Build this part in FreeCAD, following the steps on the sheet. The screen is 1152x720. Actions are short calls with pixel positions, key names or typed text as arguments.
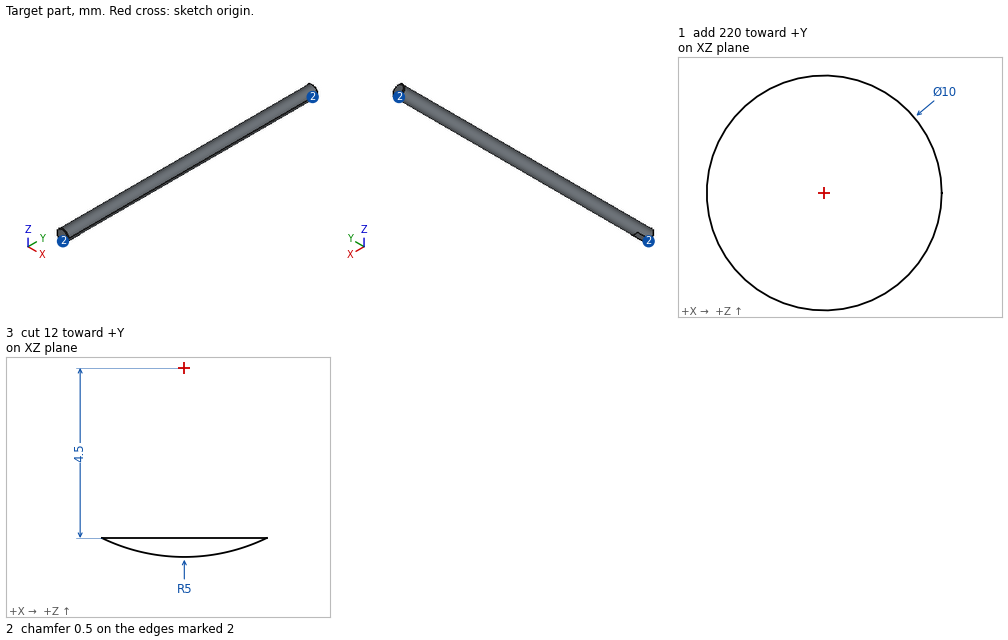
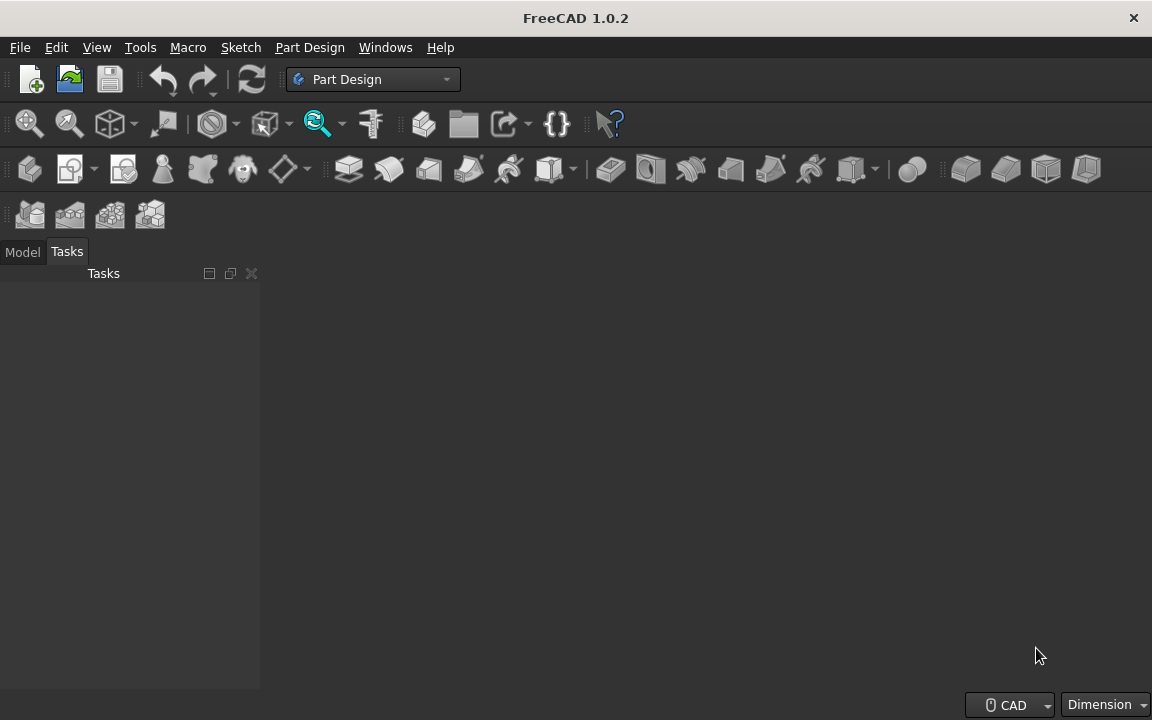
click(30, 80)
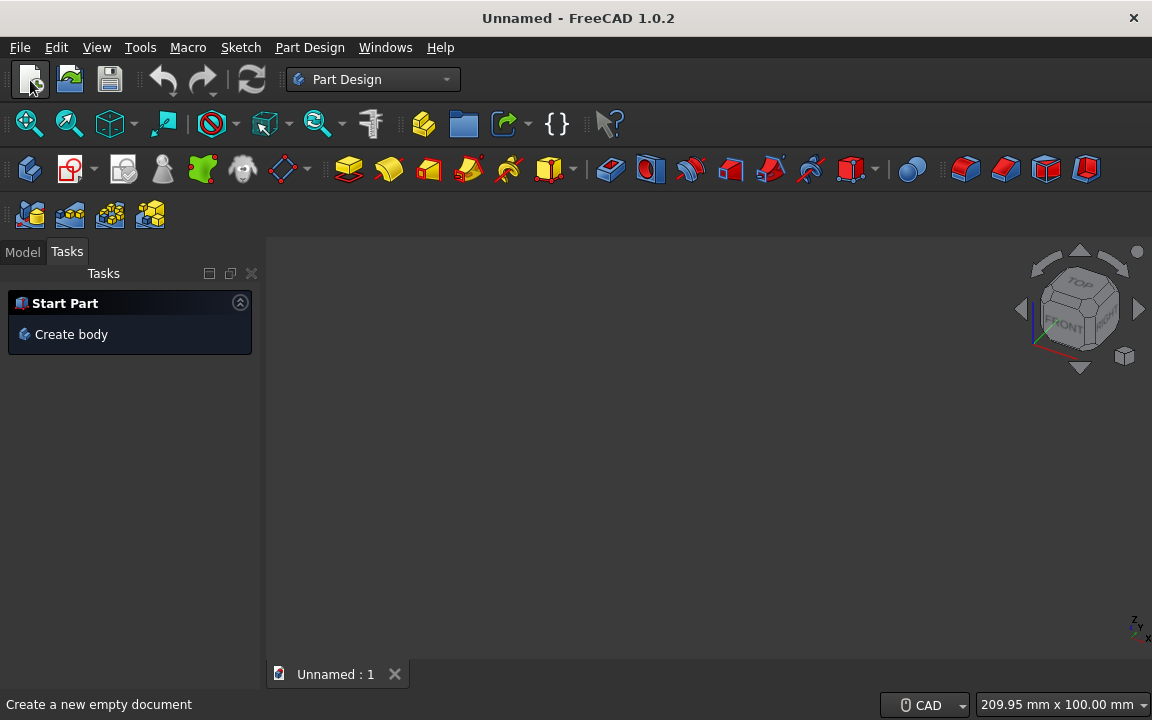
click(70, 170)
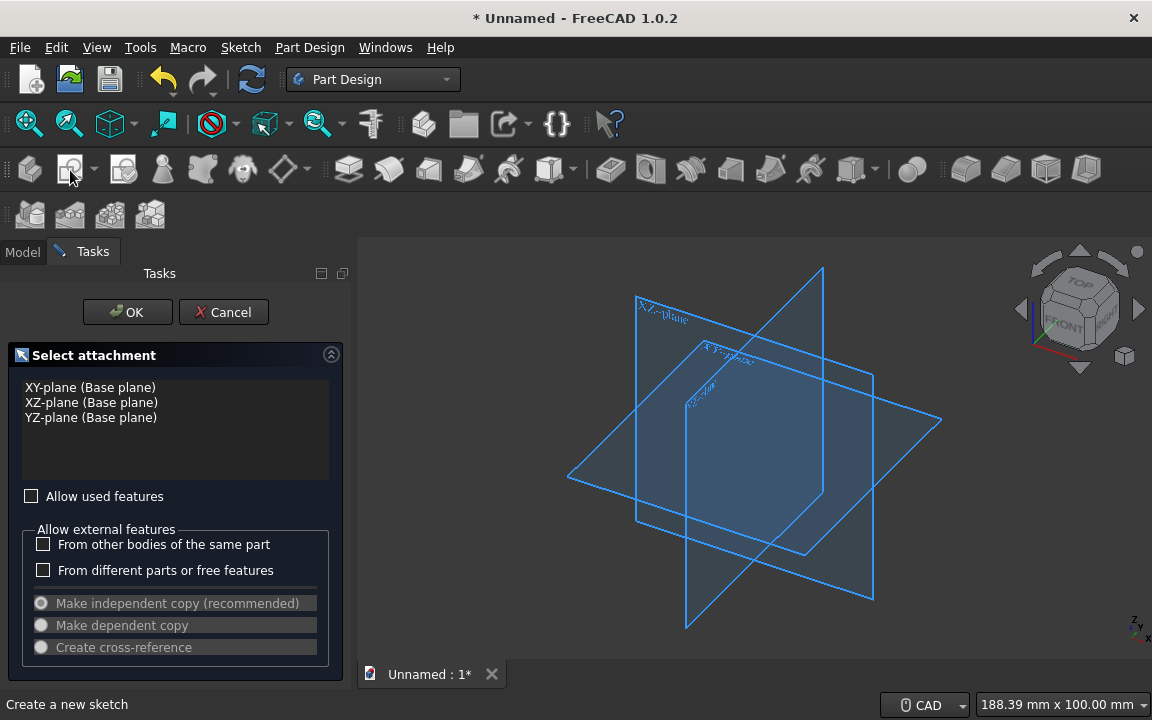
click(82, 402)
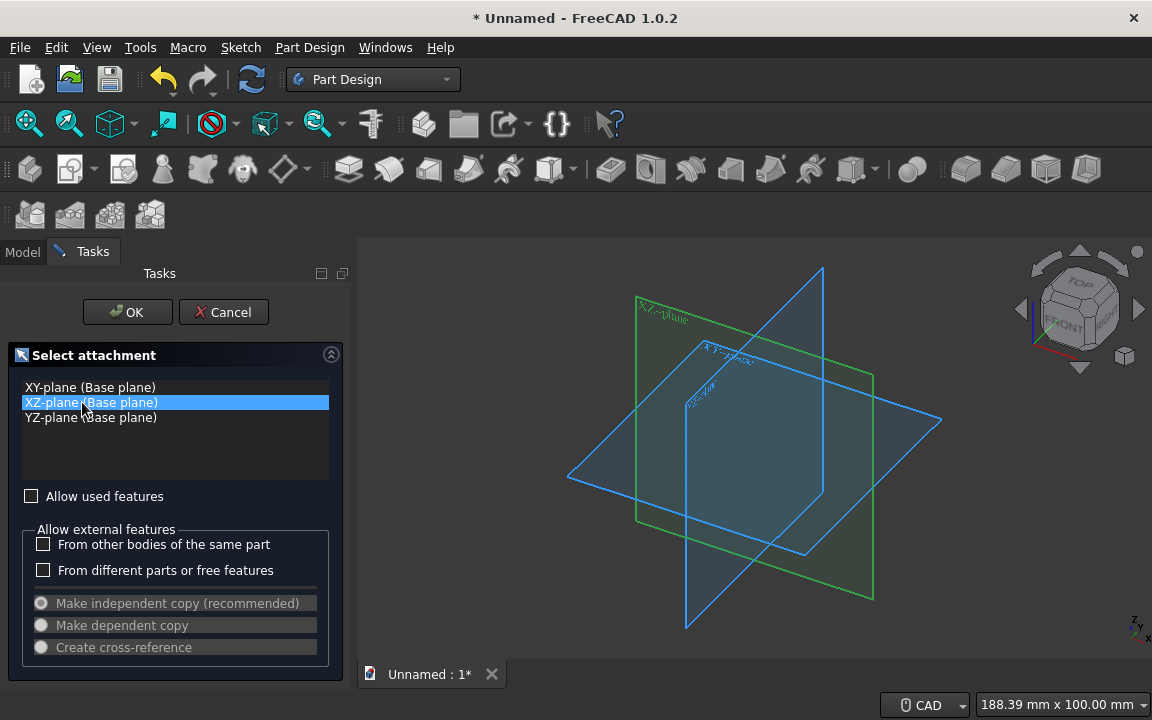
click(128, 312)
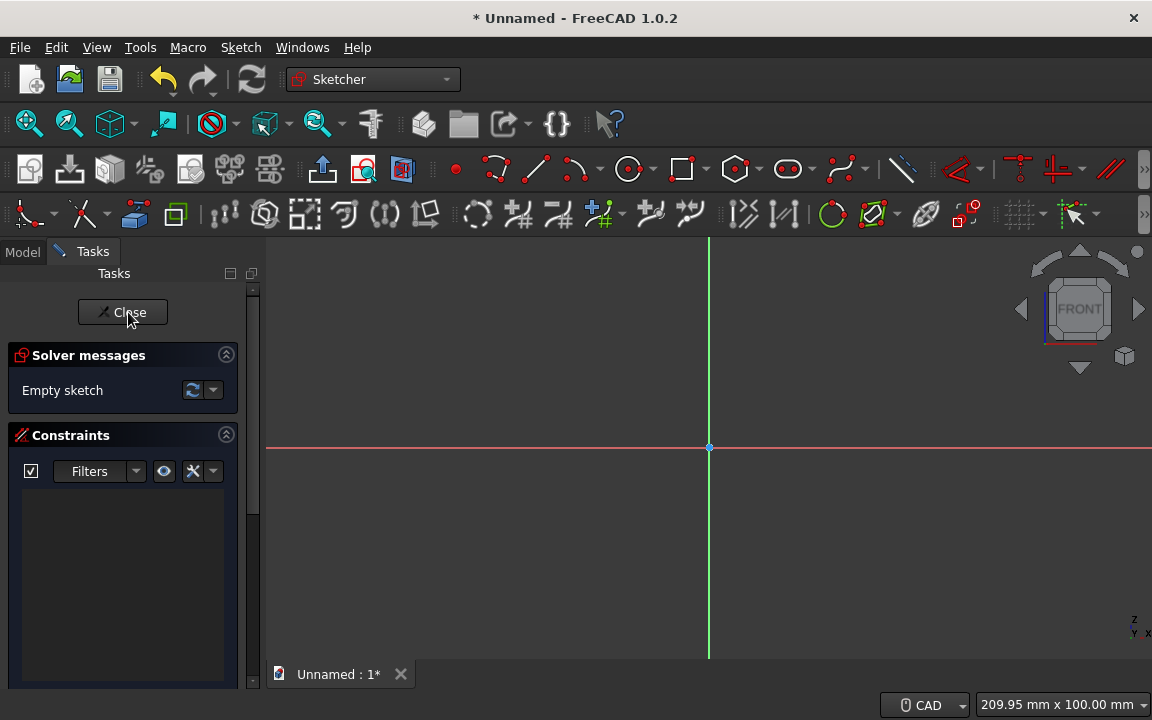
scroll(723, 448, up, 9)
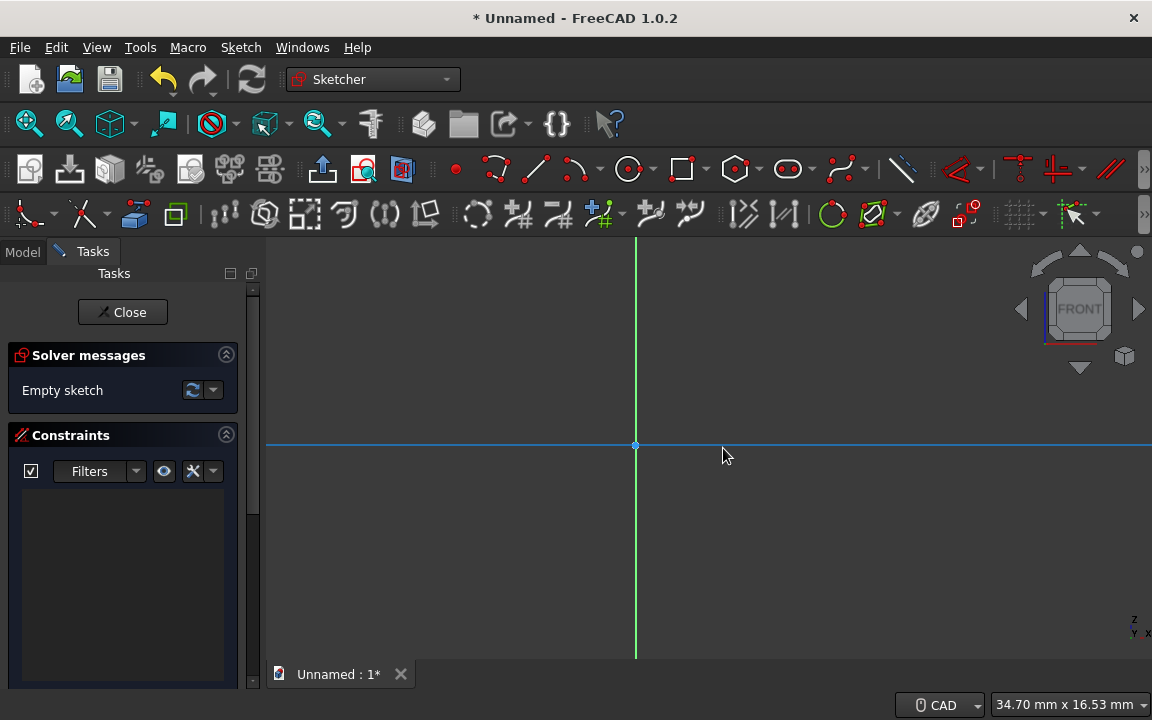
click(630, 170)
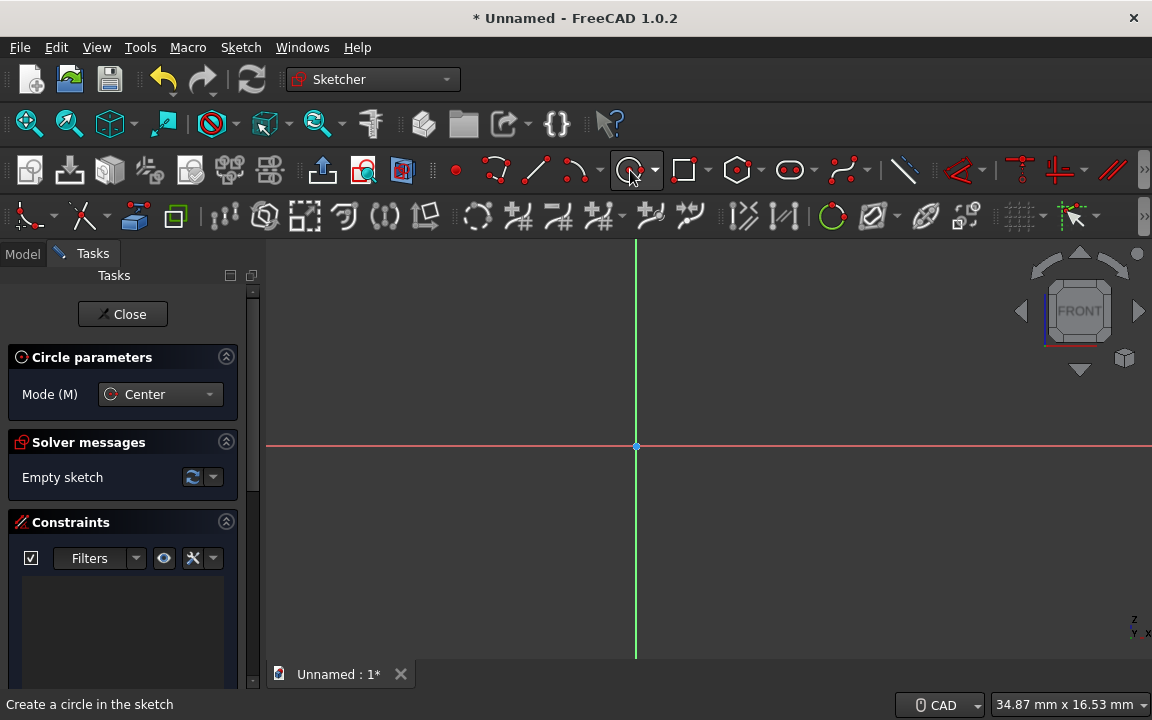
click(636, 446)
click(726, 357)
key(Escape)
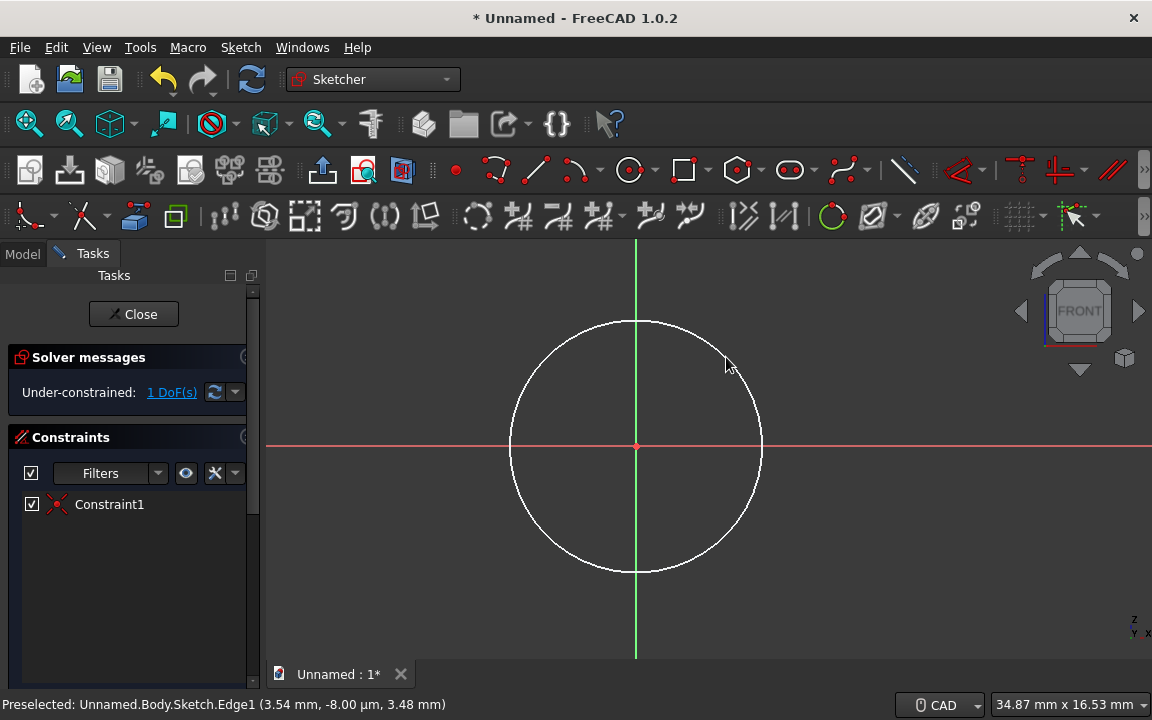
click(958, 170)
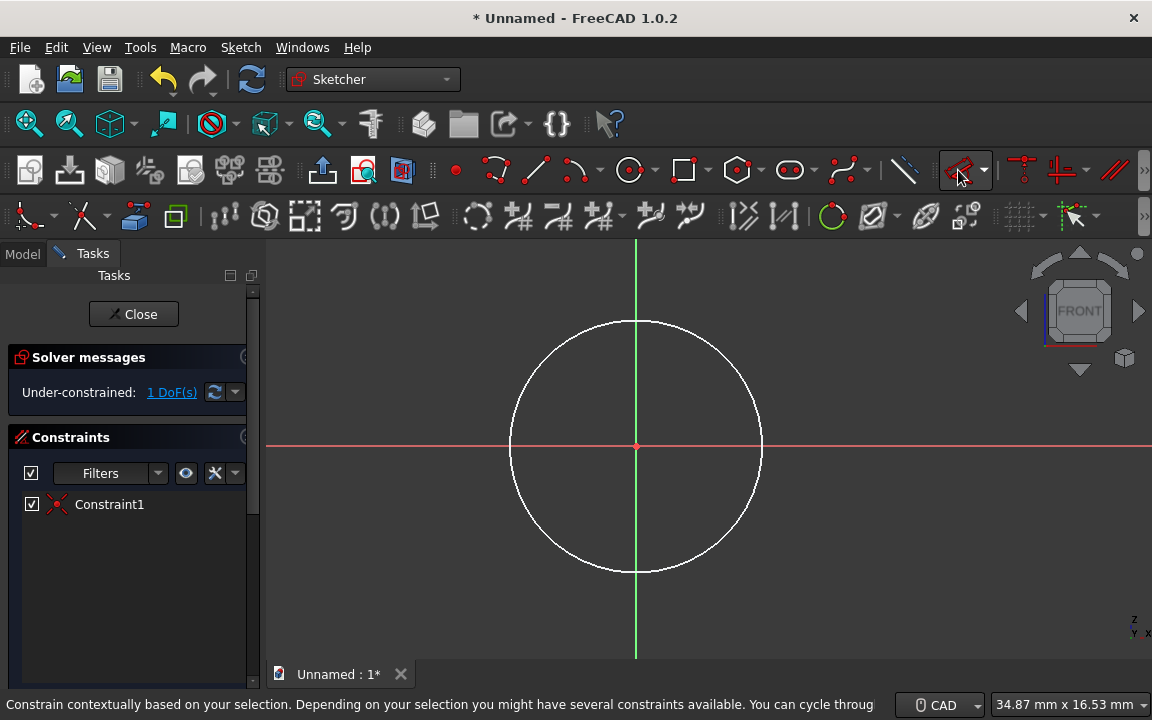
click(725, 357)
click(748, 334)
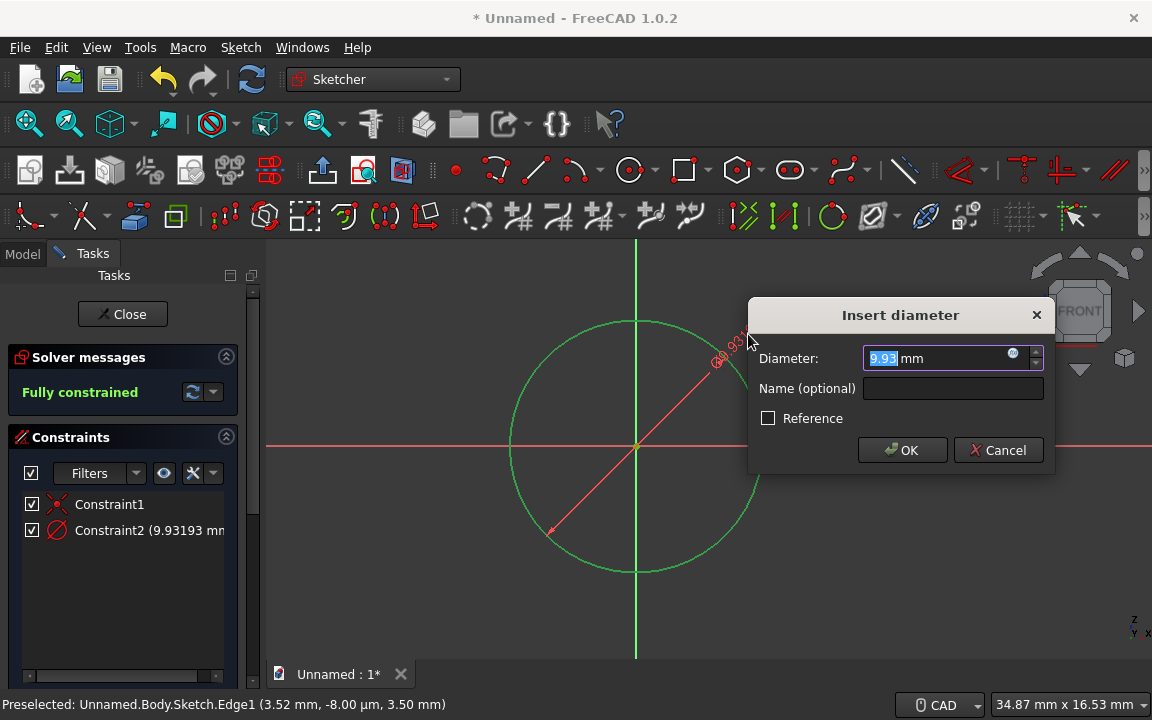
text(10)
key(Return)
key(Escape)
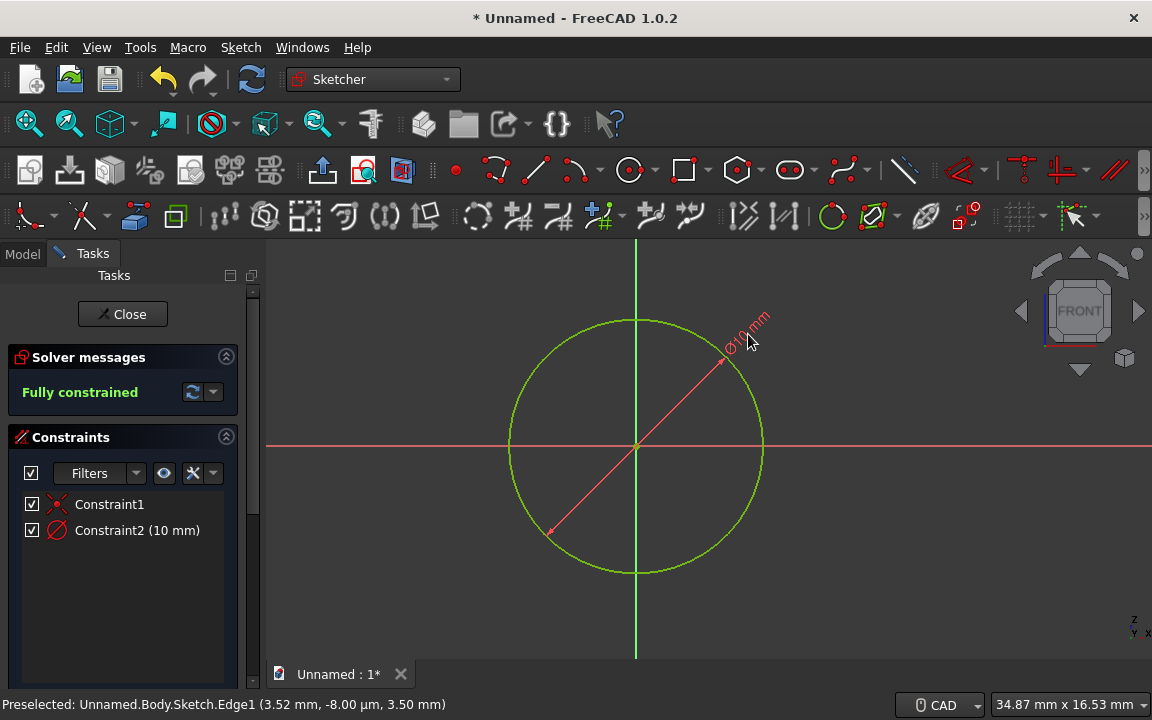
click(123, 314)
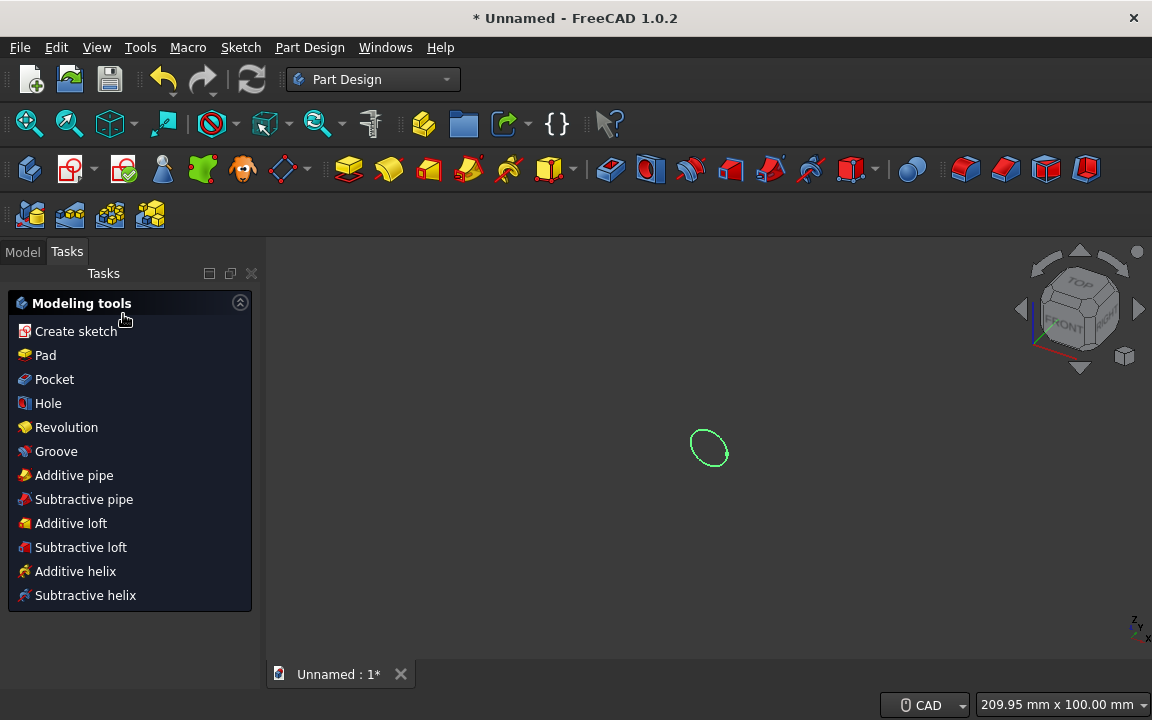
click(350, 170)